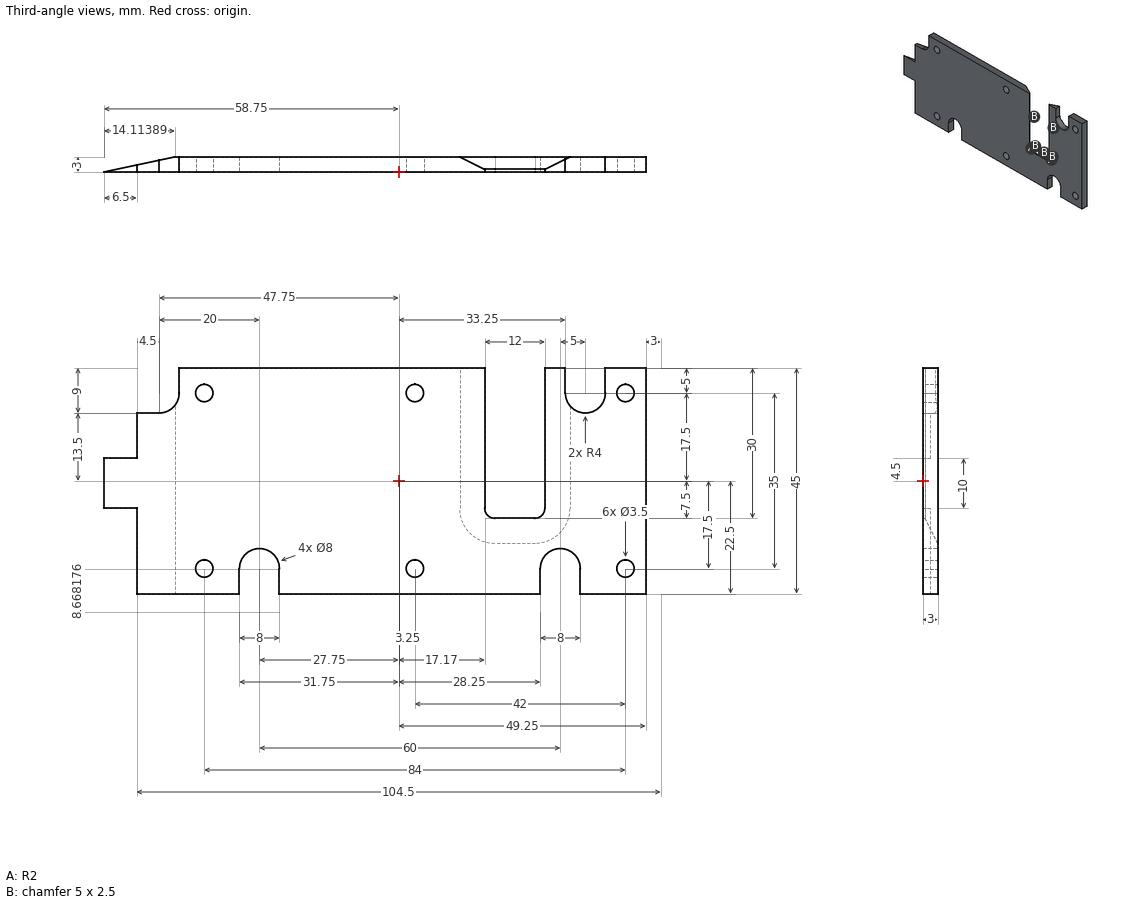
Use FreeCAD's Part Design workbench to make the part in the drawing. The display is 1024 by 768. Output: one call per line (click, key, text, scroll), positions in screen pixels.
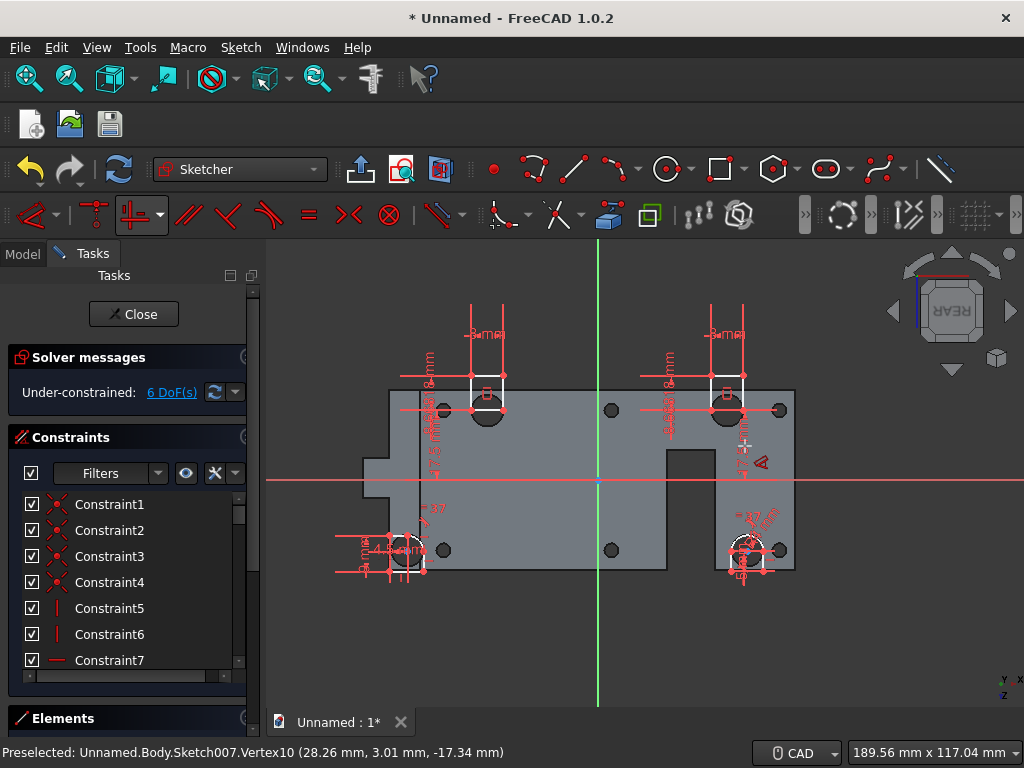
click(731, 551)
click(765, 500)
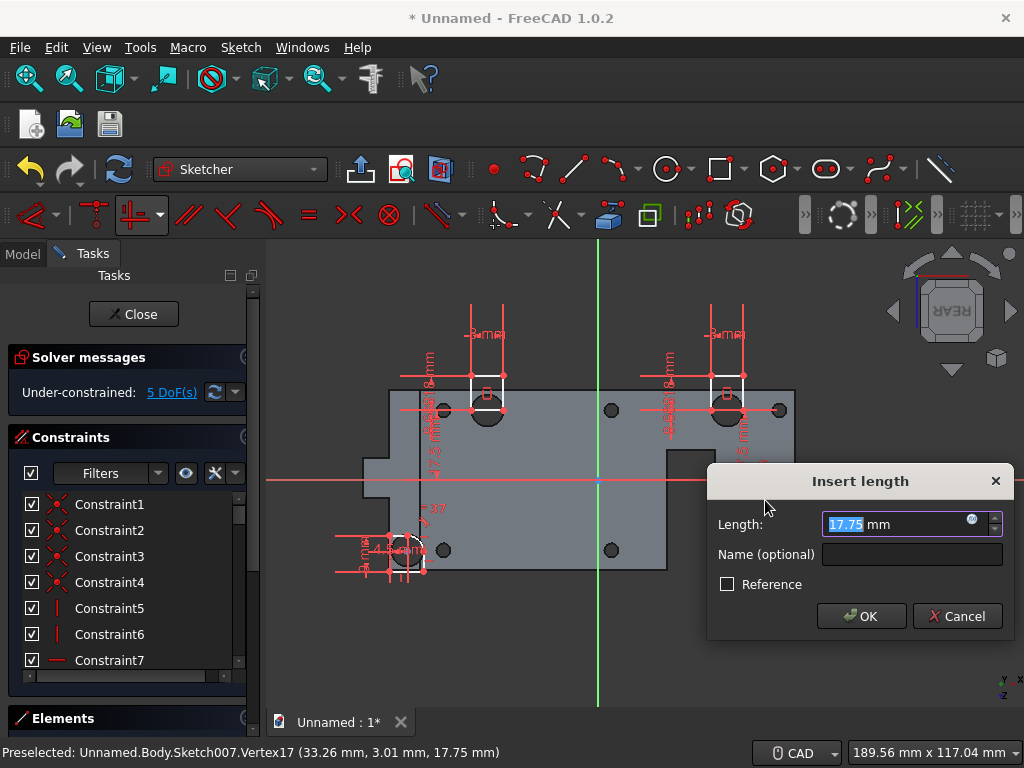
text(17.5)
key(Return)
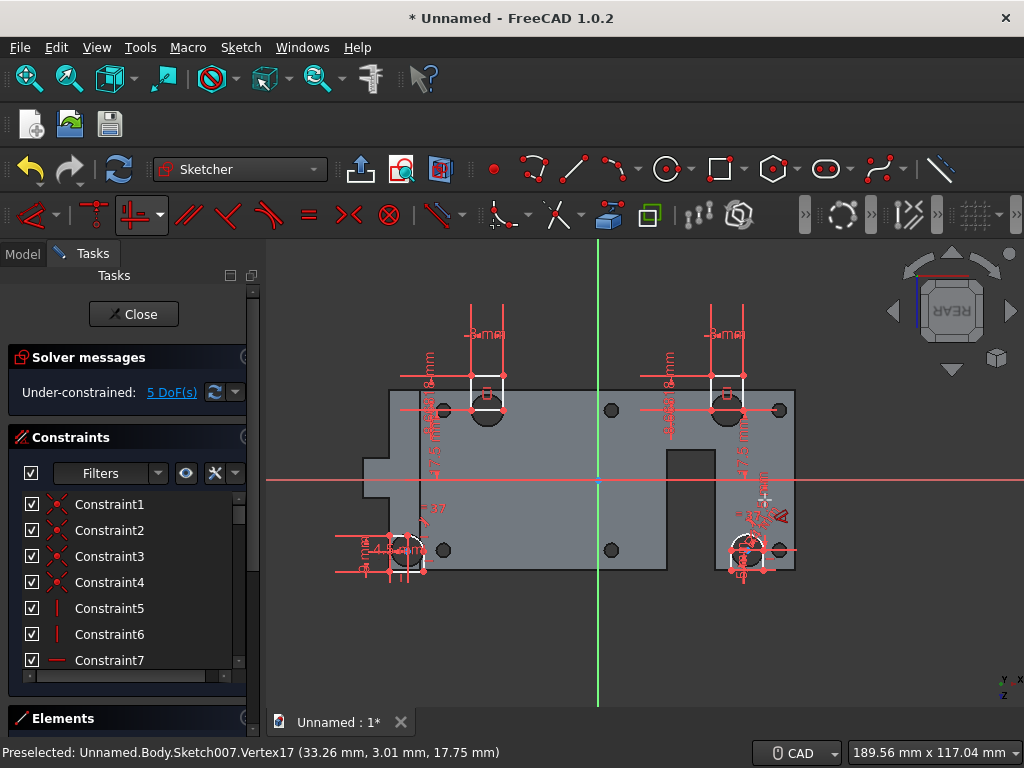
click(408, 536)
click(374, 508)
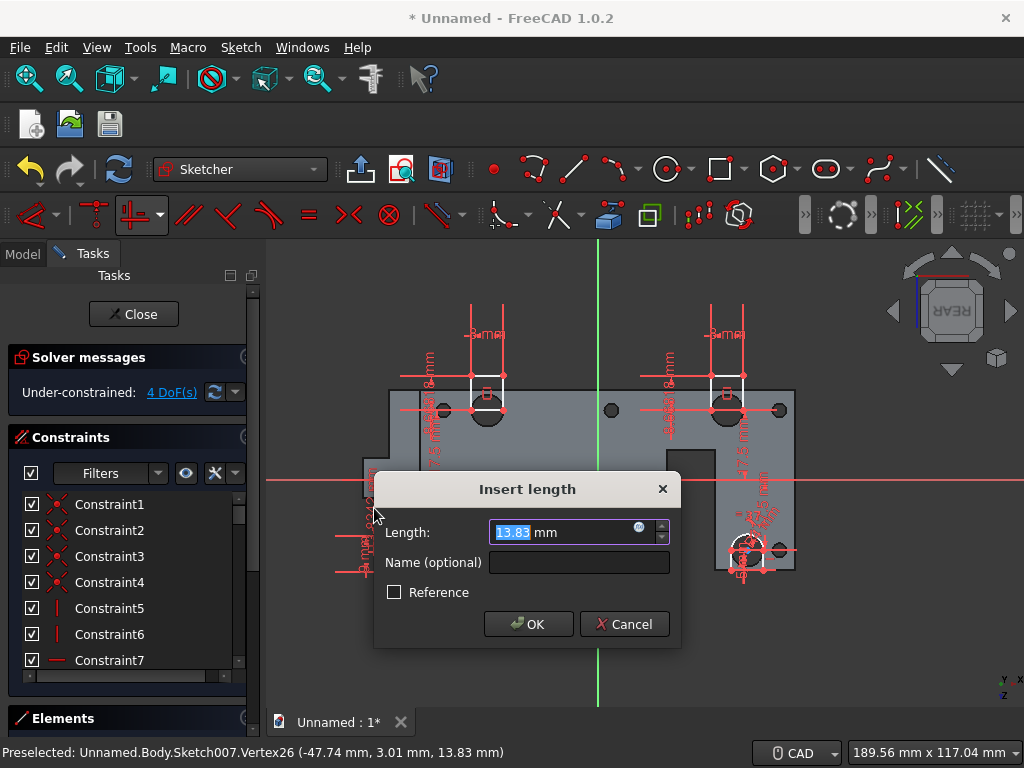
text(13.5)
key(Return)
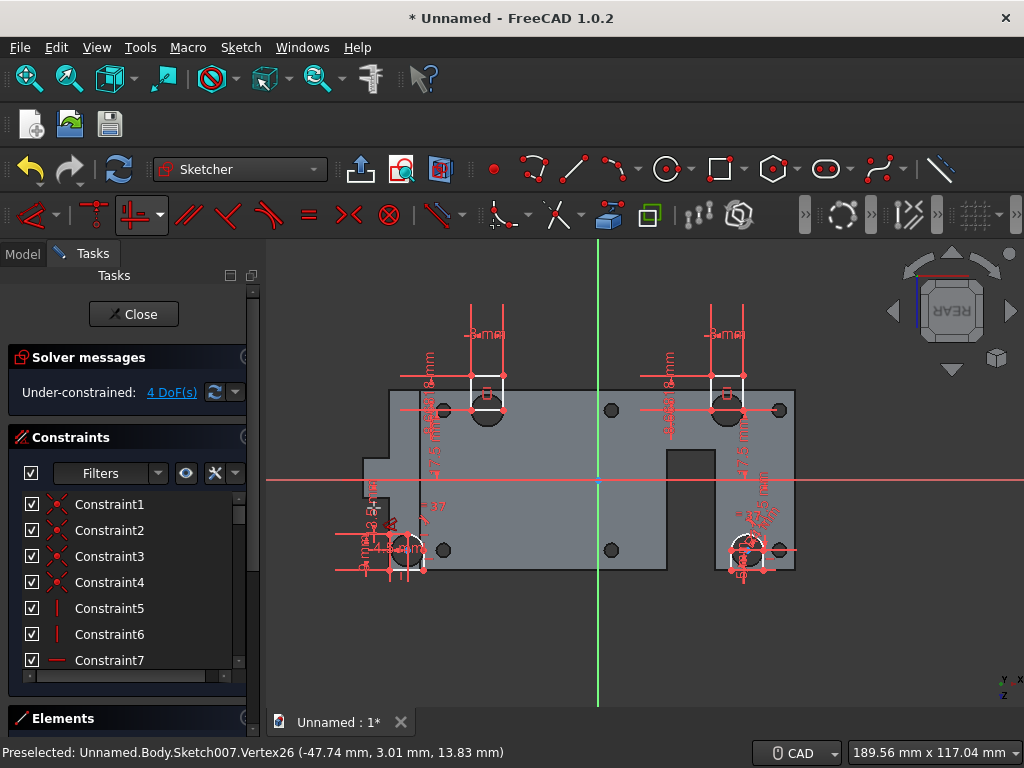
click(471, 376)
click(535, 342)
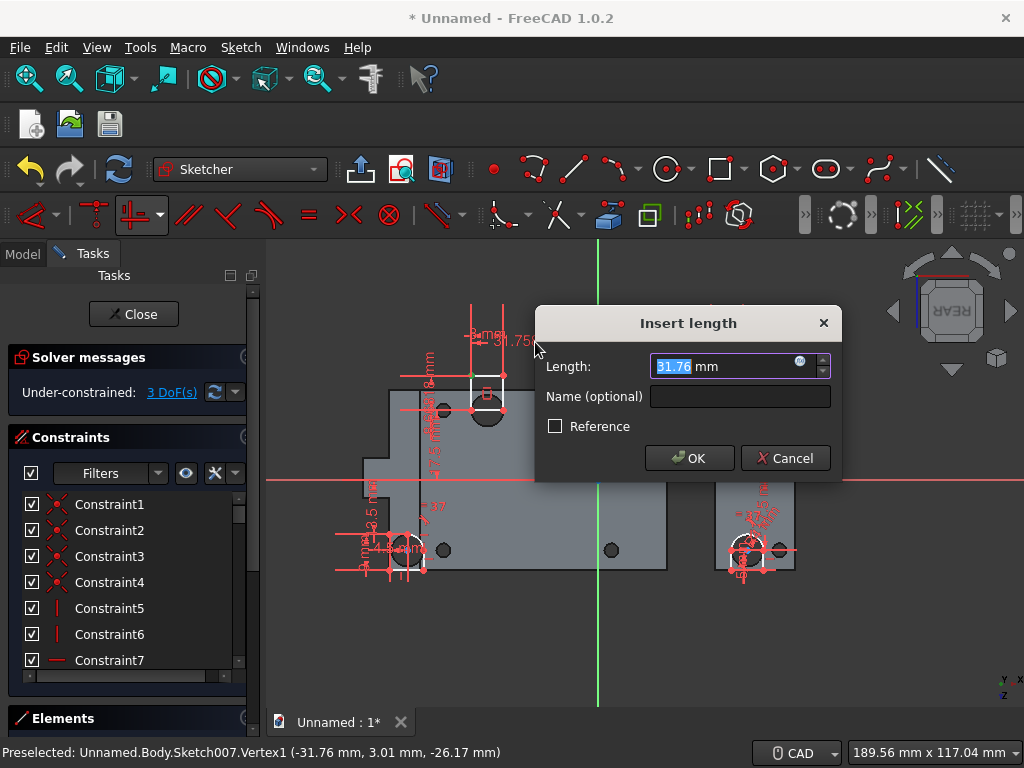
text(31.75)
key(Return)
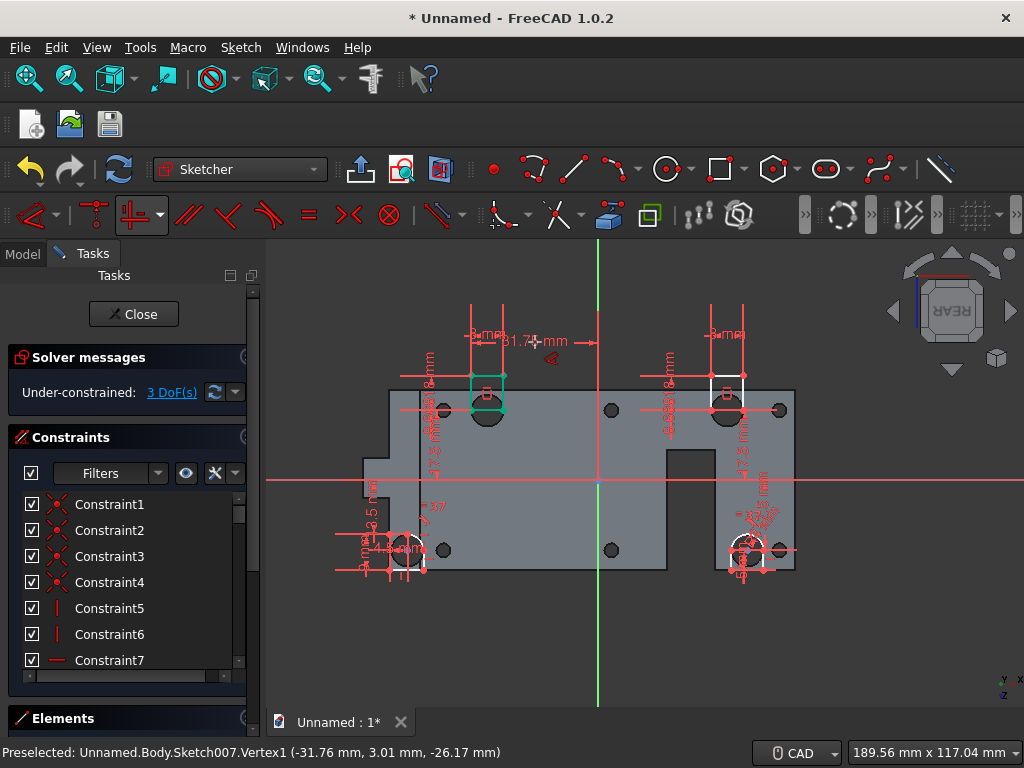
click(711, 376)
click(655, 342)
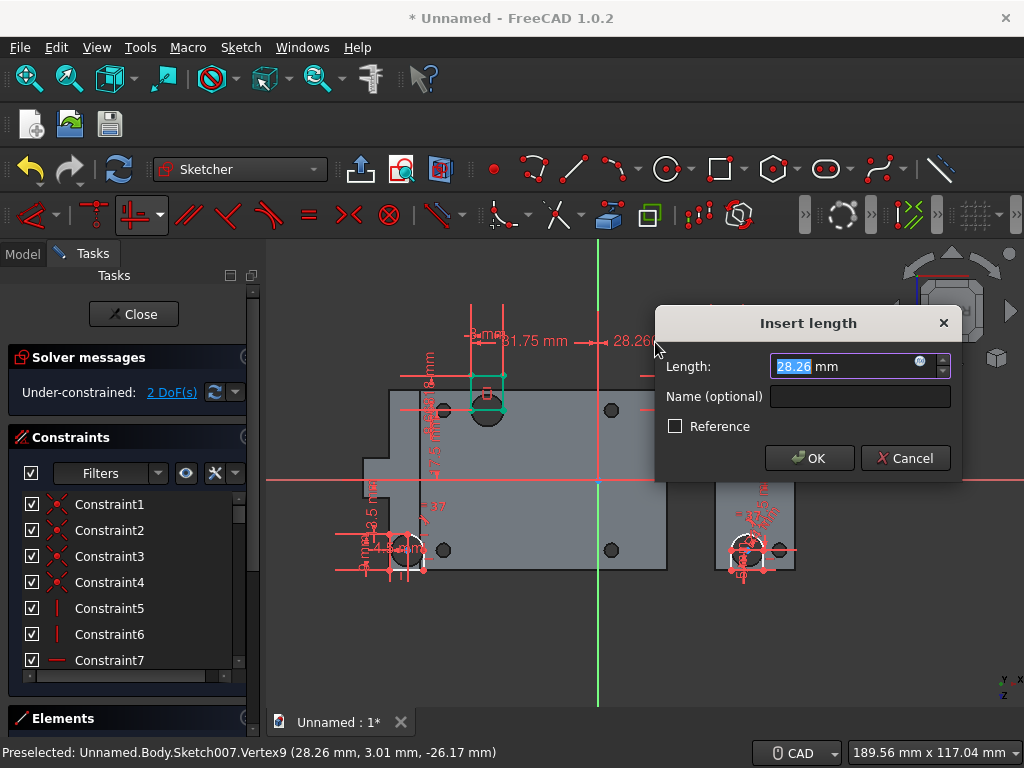
text(28.25)
key(Return)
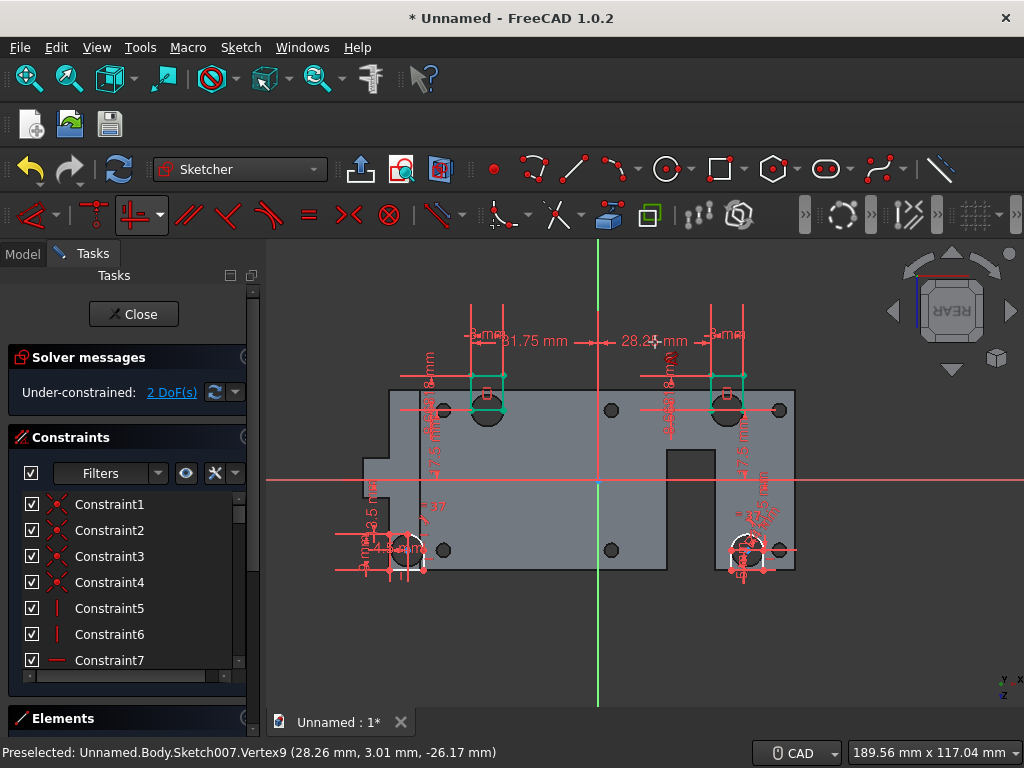
click(731, 550)
click(665, 584)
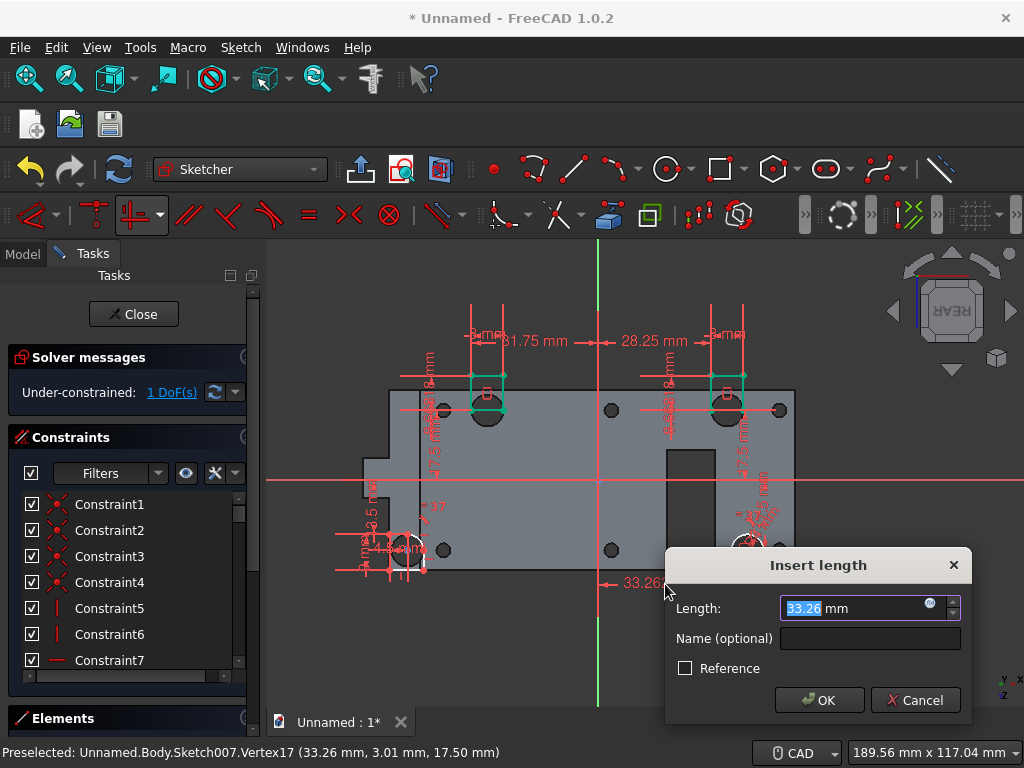
text(33.25)
key(Return)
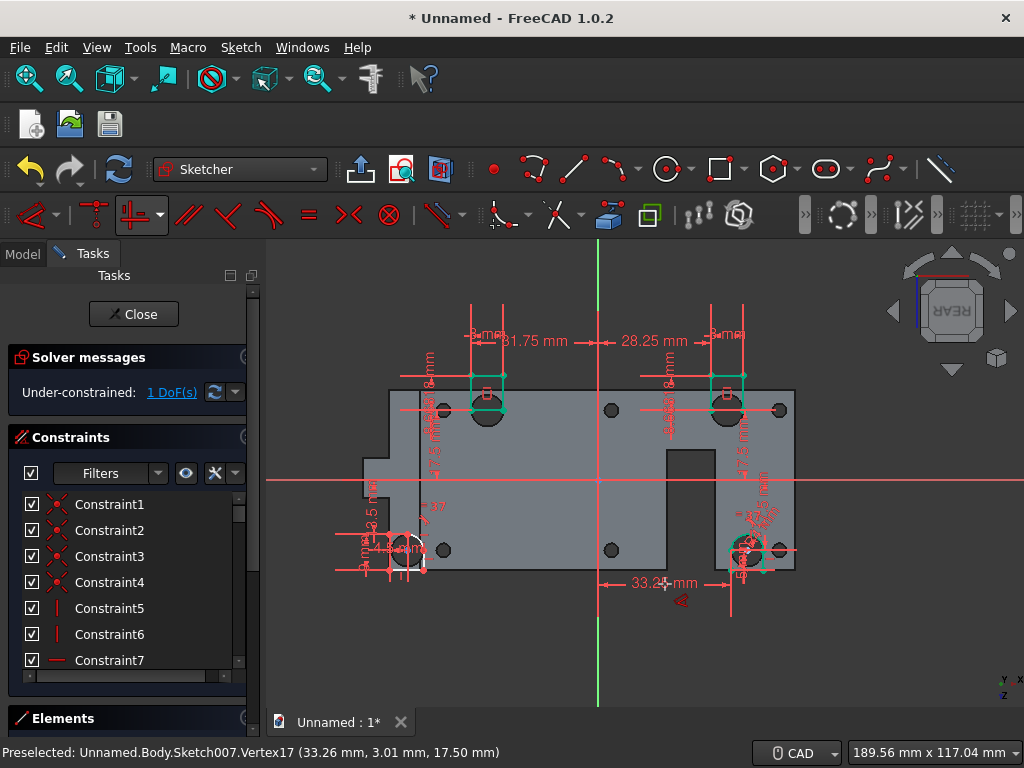
click(408, 534)
click(503, 568)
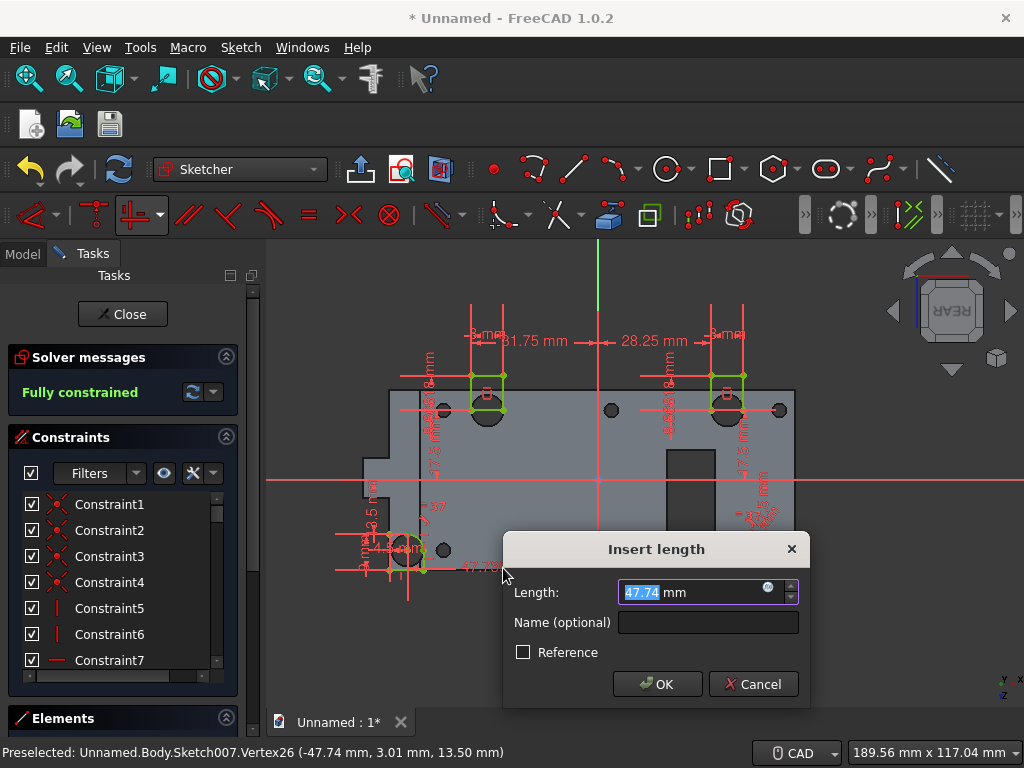
text(47.75)
key(Return)
key(Escape)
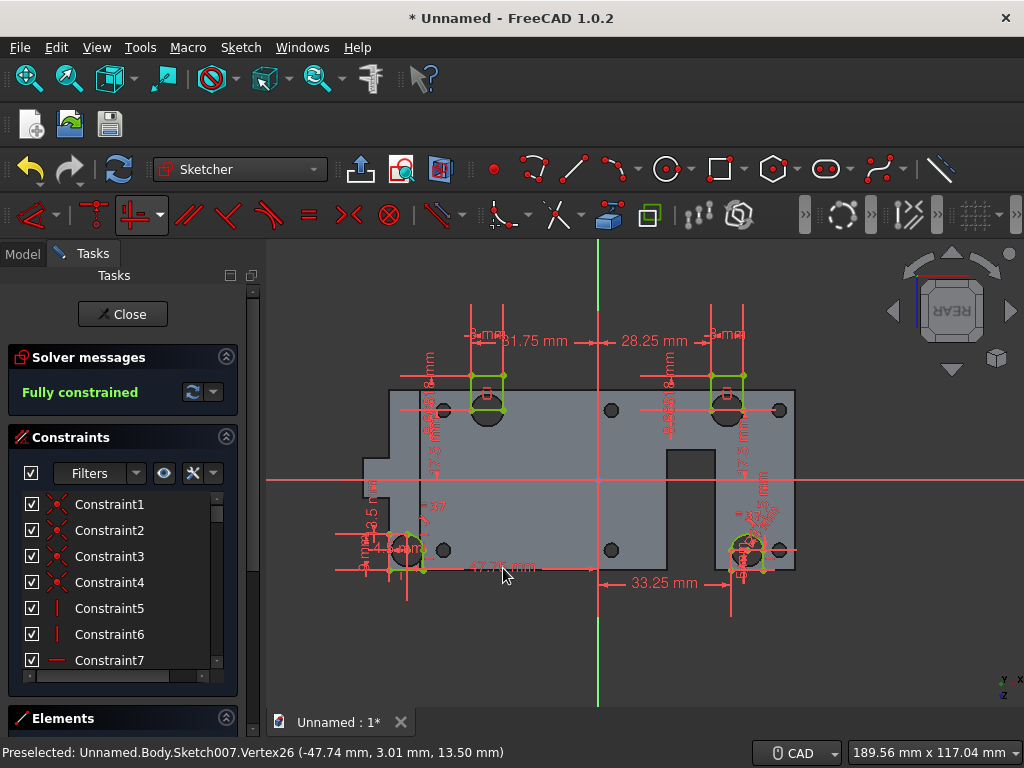
click(123, 314)